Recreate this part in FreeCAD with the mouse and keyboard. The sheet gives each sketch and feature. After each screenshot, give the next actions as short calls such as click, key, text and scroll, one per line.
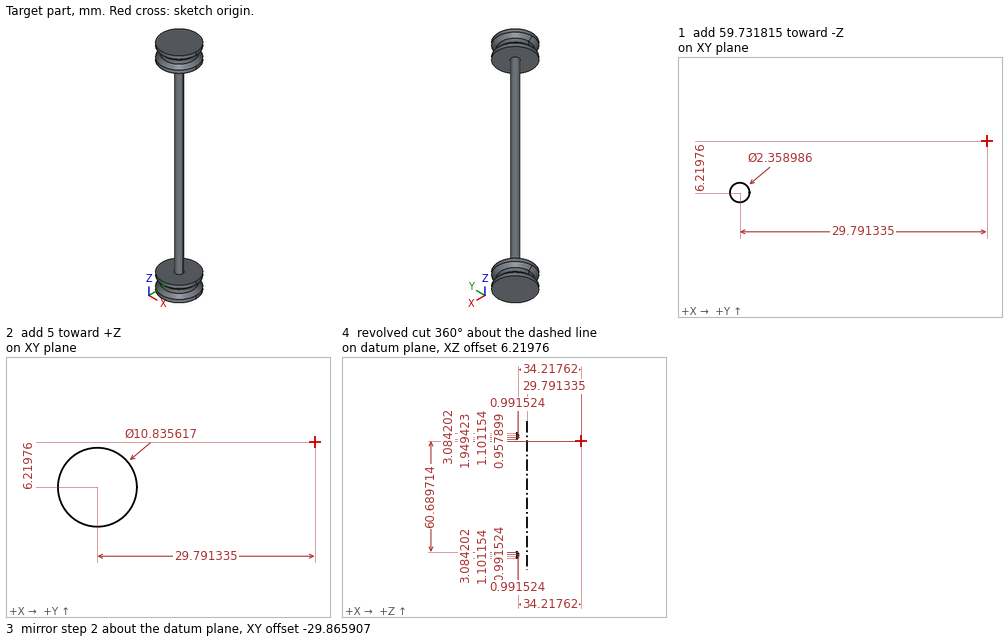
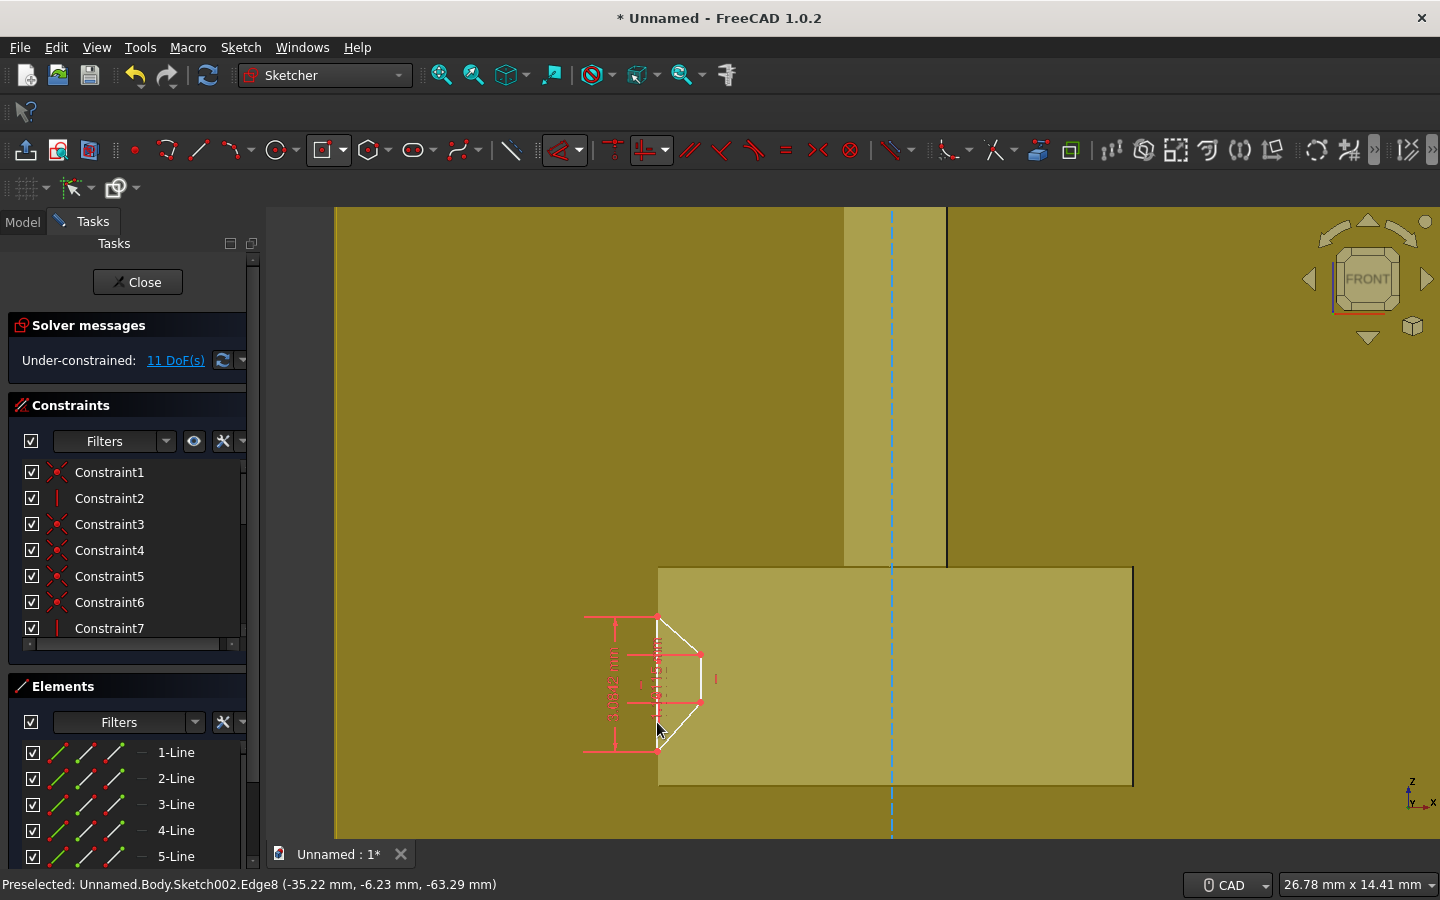
scroll(704, 681, down, 11)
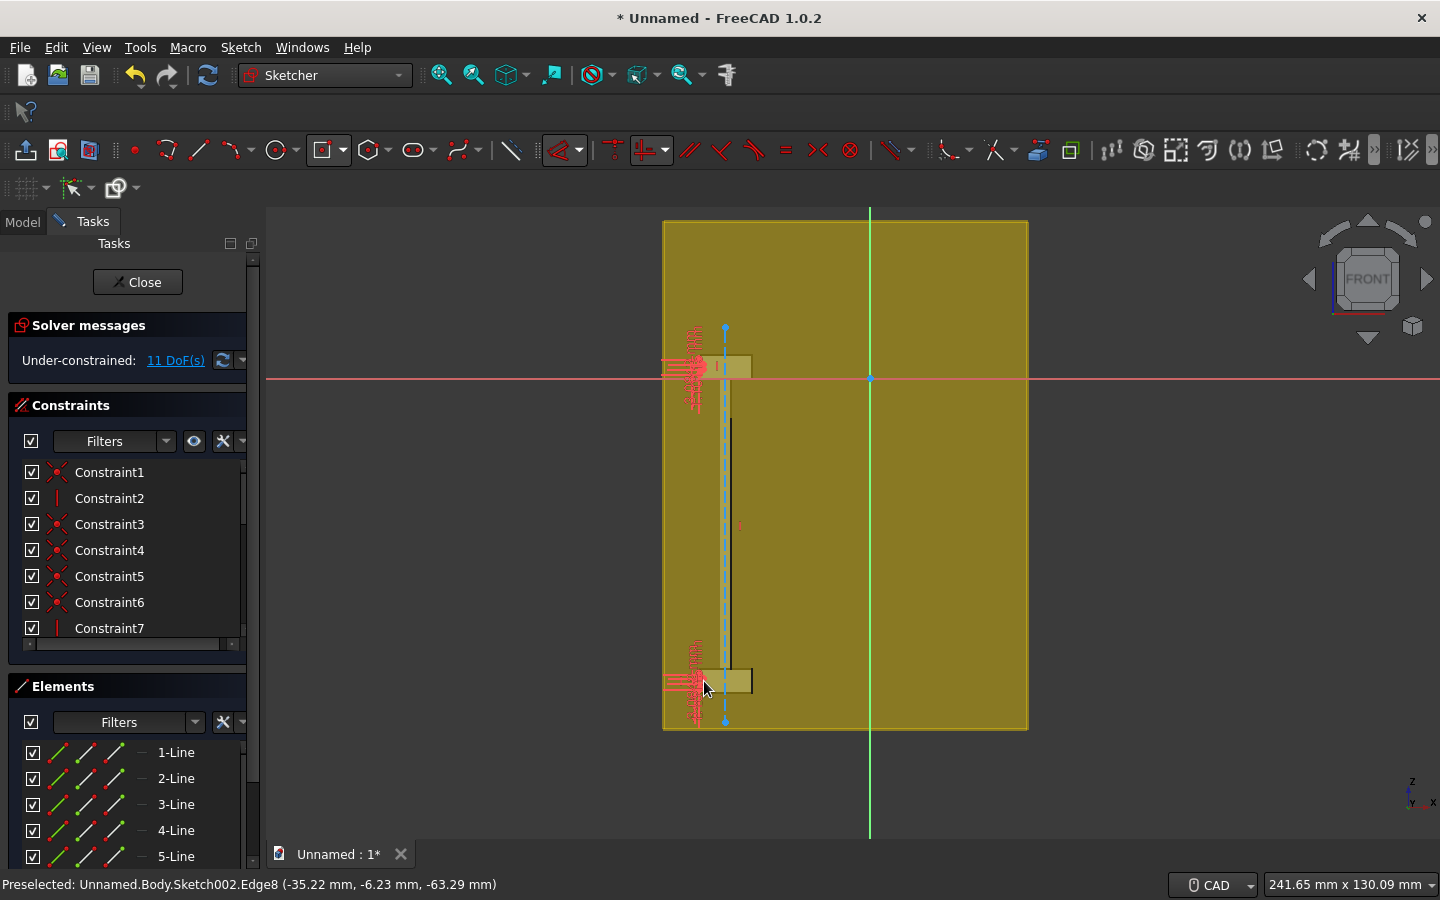
scroll(704, 370, up, 5)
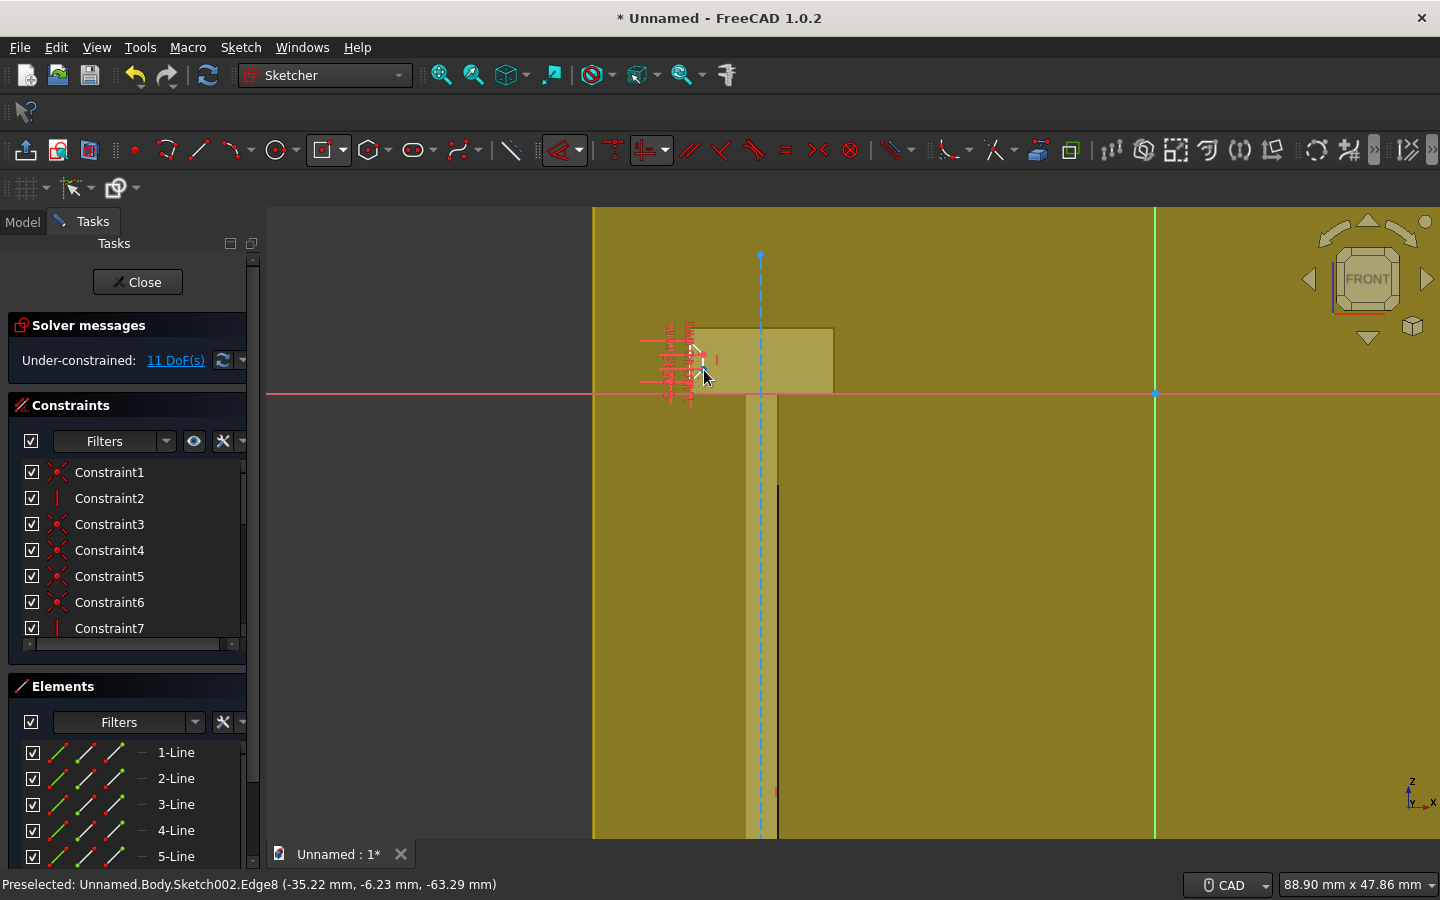
click(703, 369)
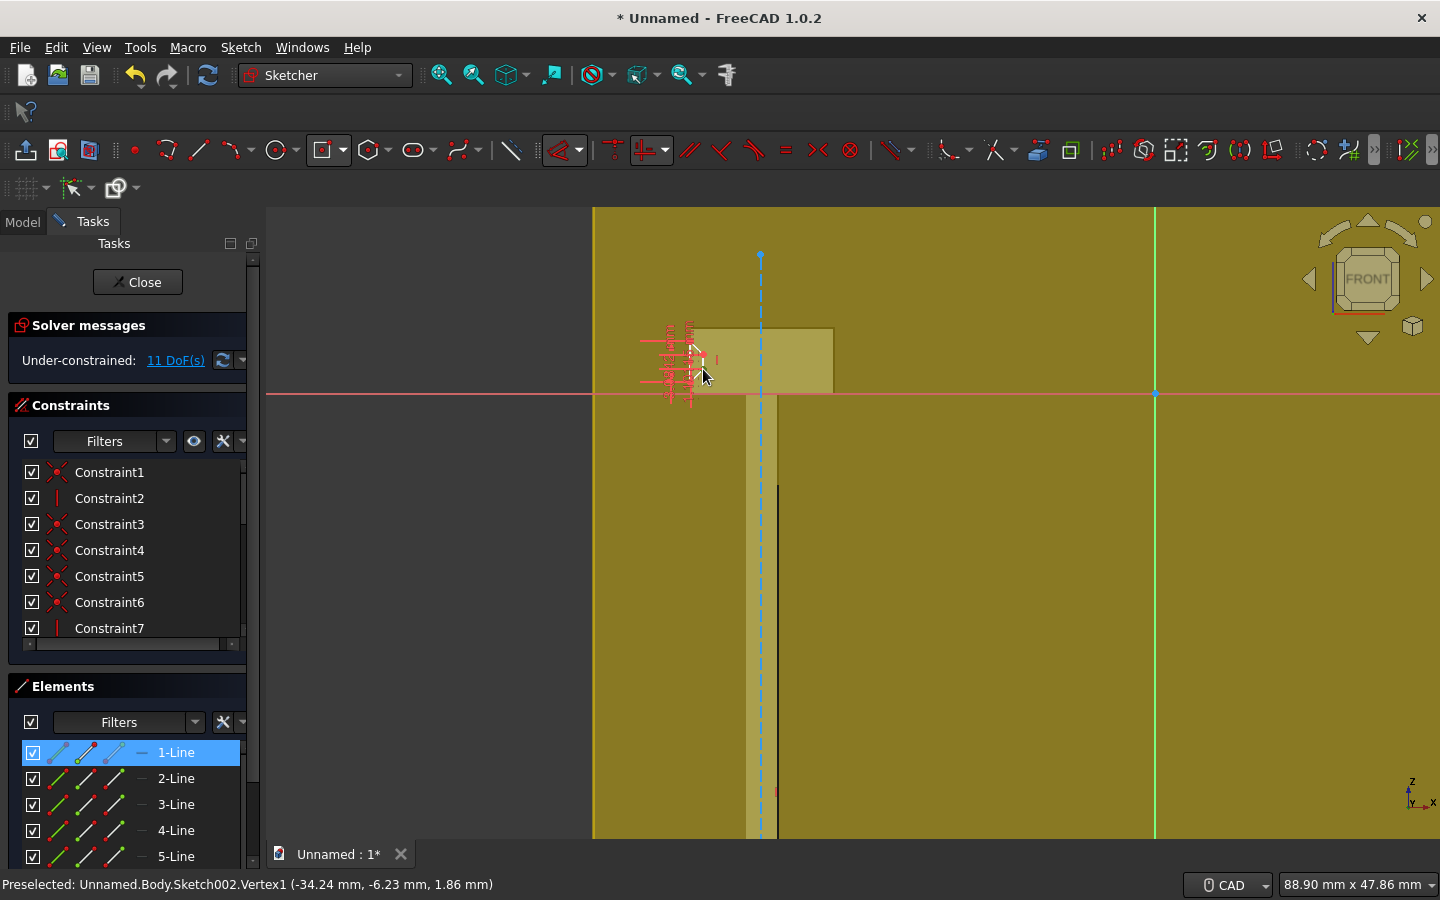
key(l)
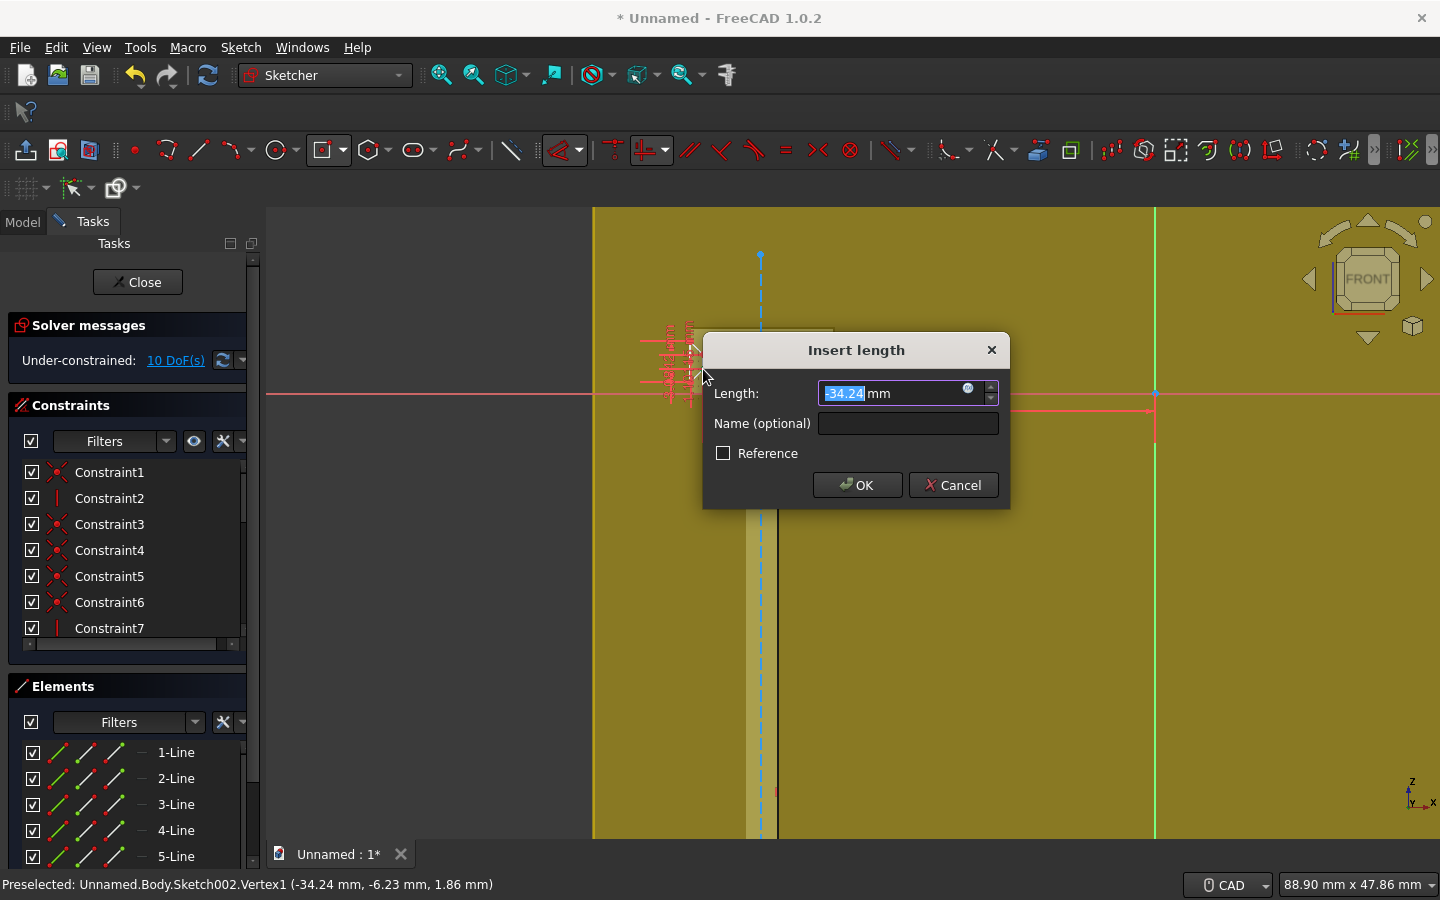
text(-34.21762)
key(Return)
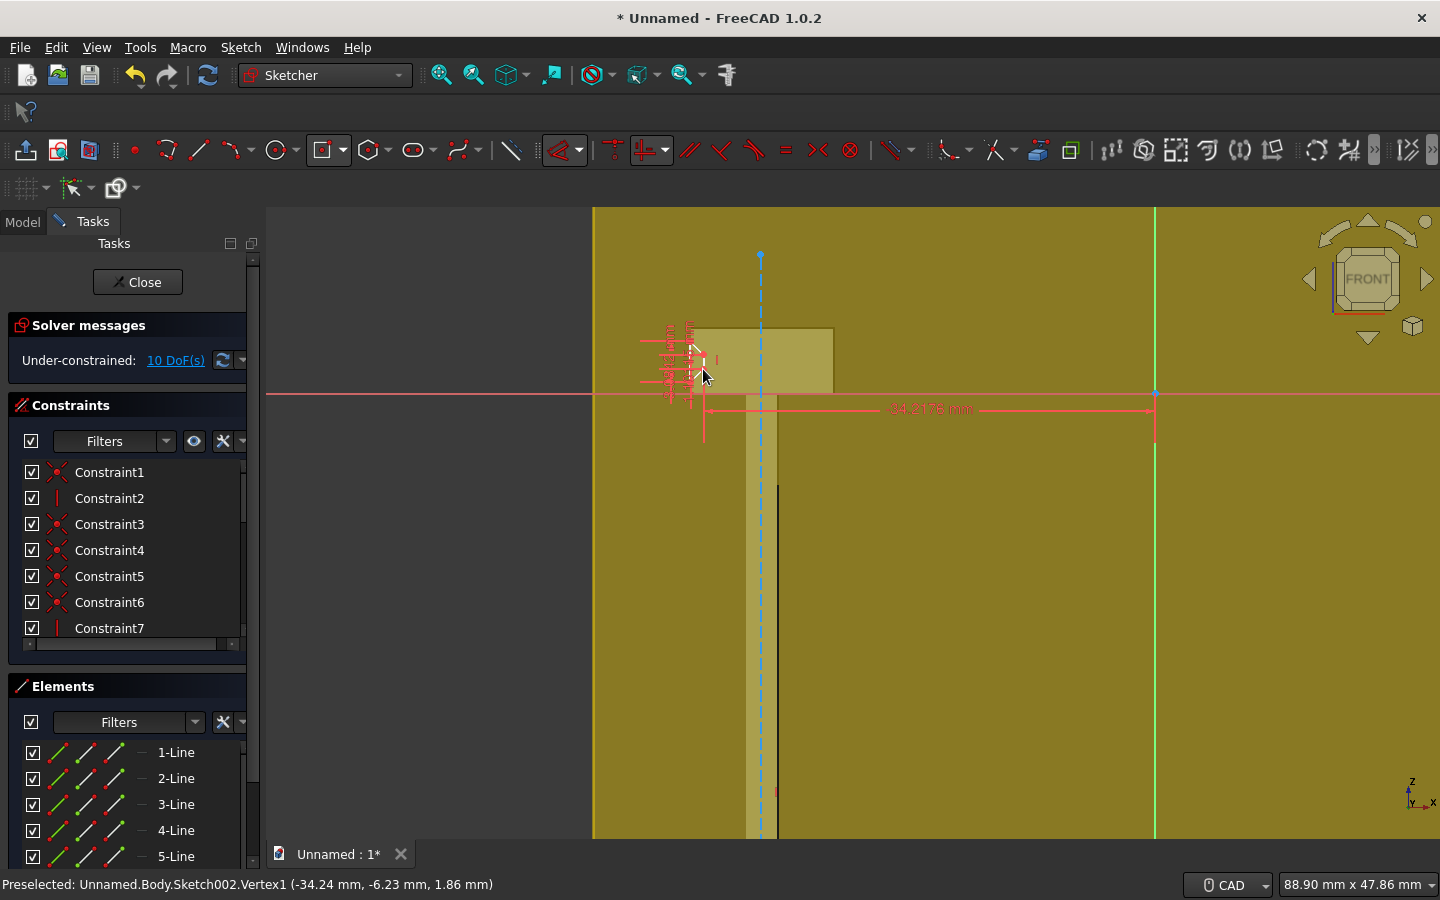
scroll(704, 369, up, 3)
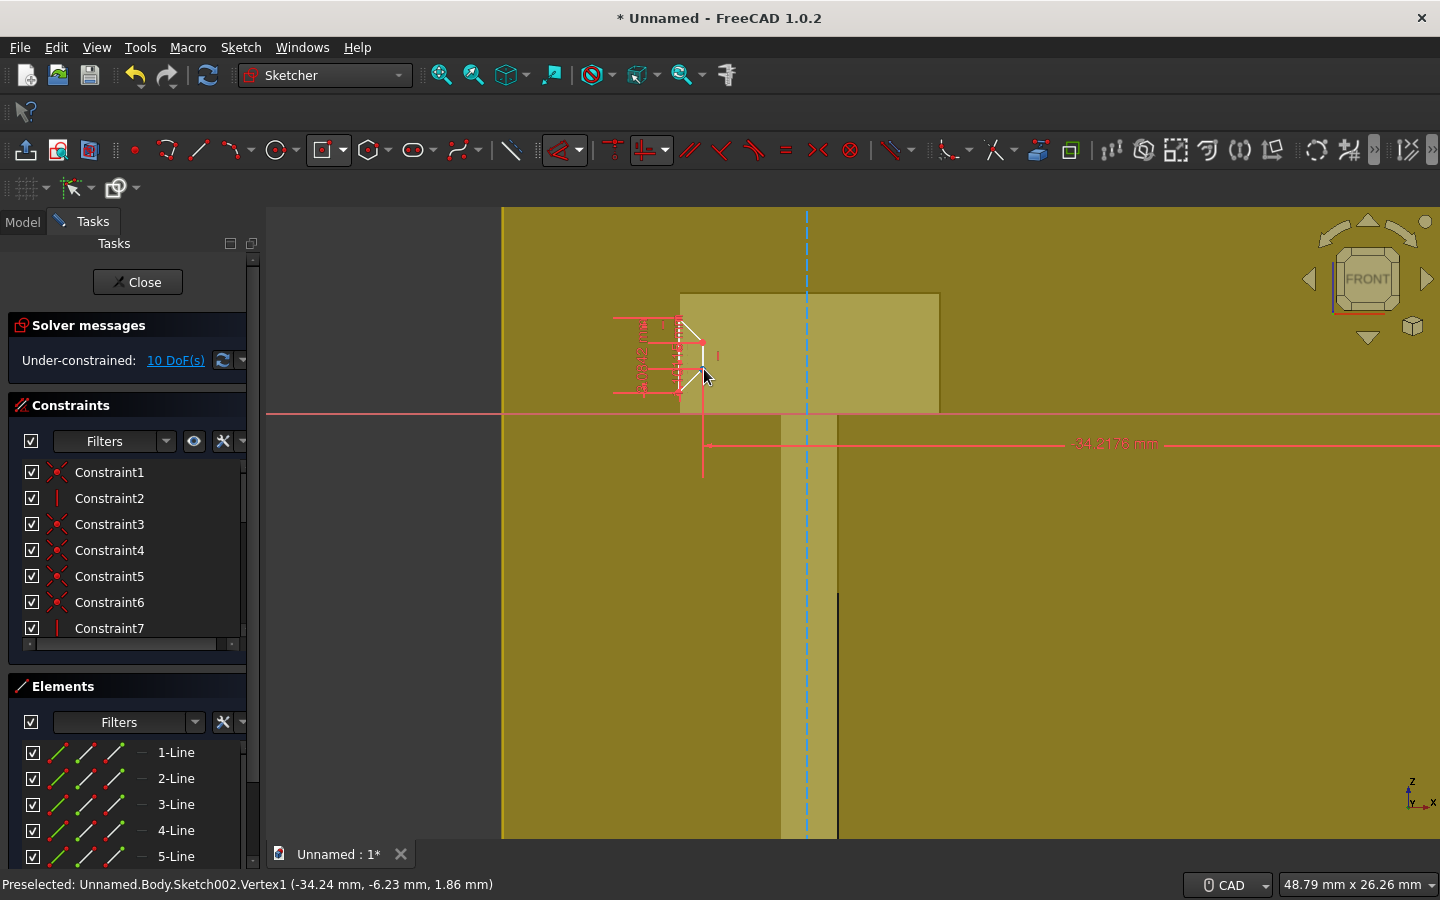
click(703, 369)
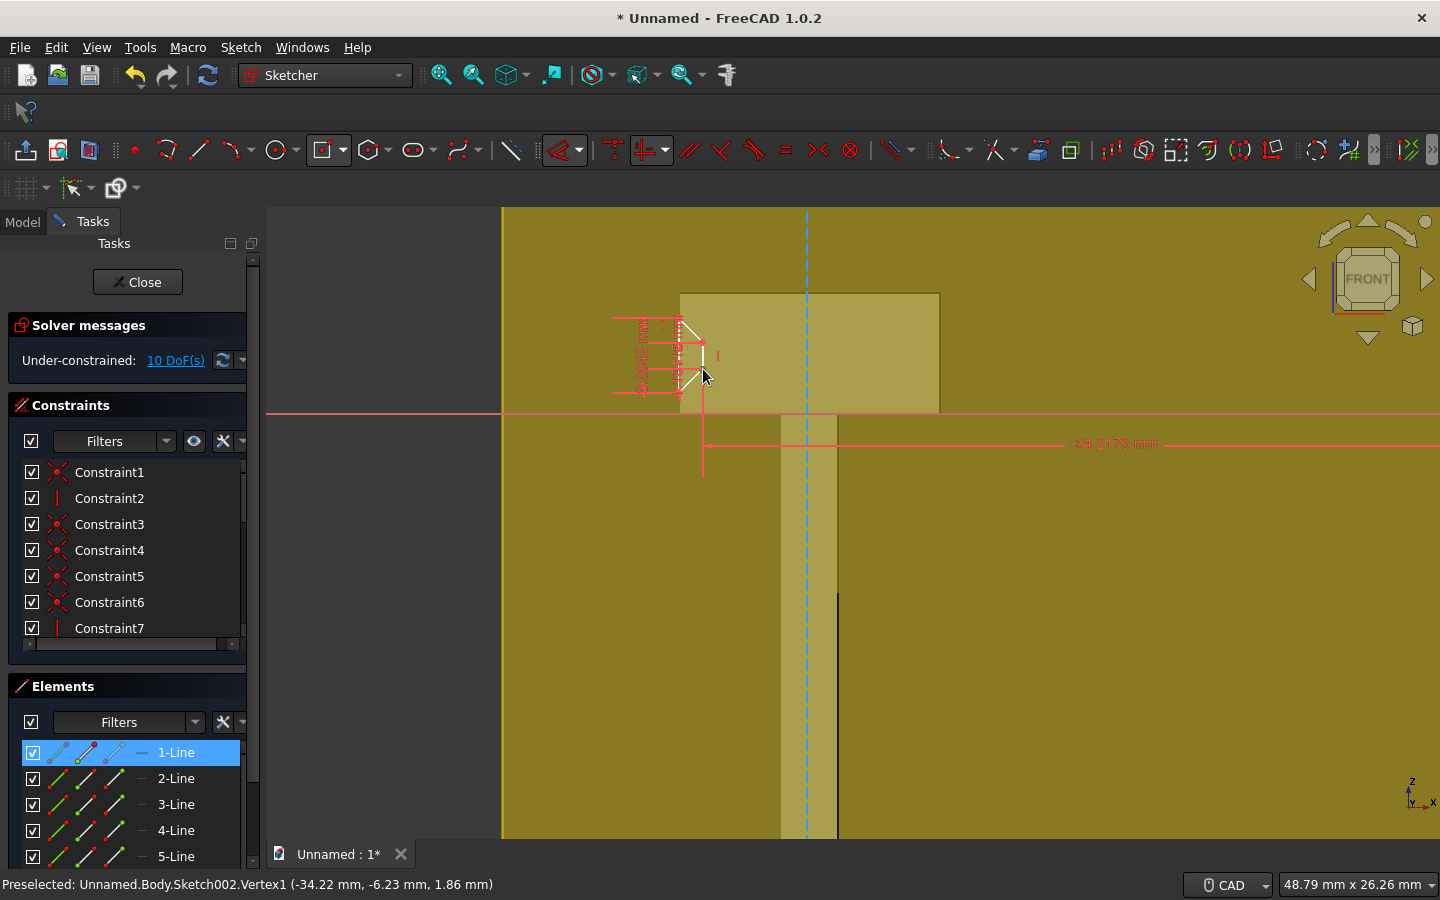
key(i)